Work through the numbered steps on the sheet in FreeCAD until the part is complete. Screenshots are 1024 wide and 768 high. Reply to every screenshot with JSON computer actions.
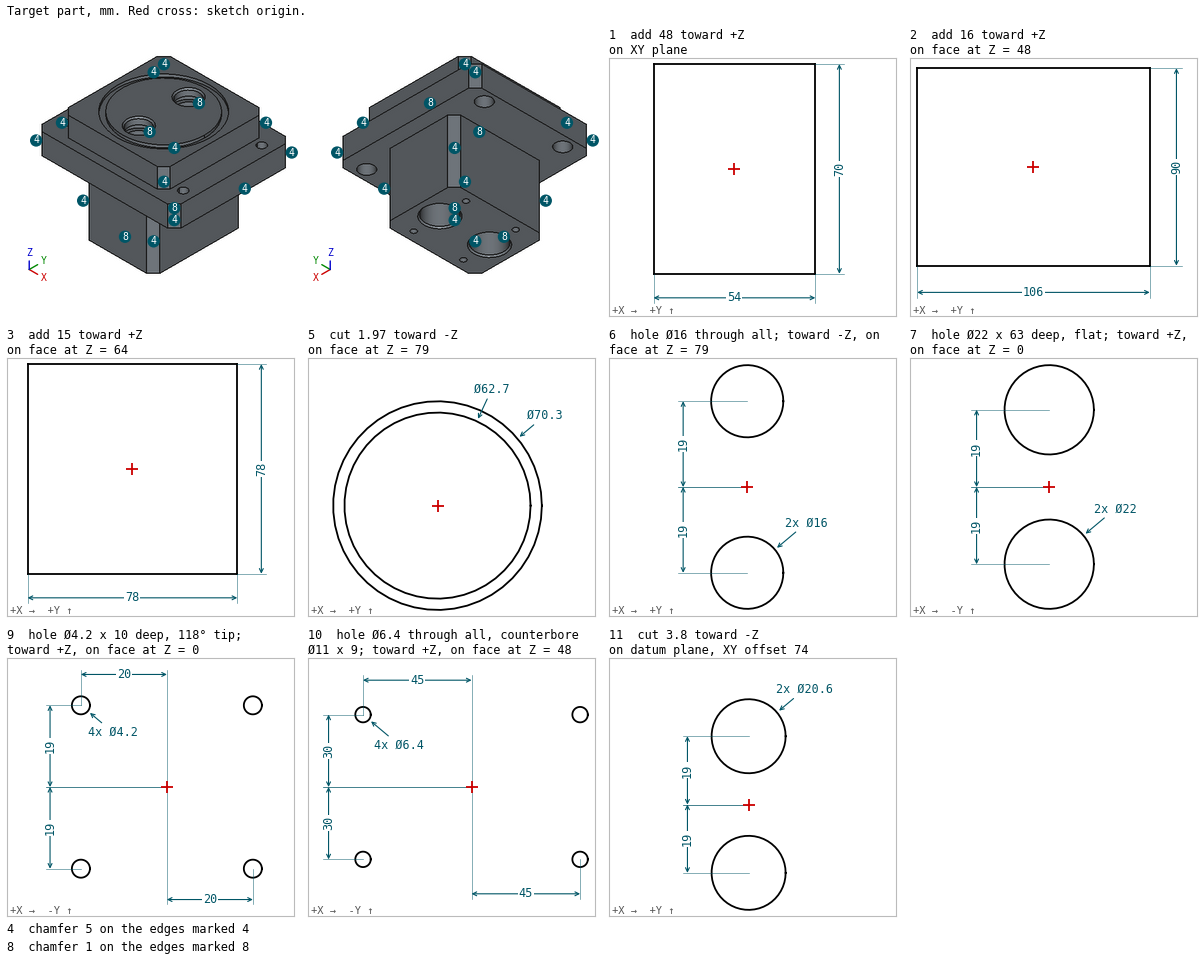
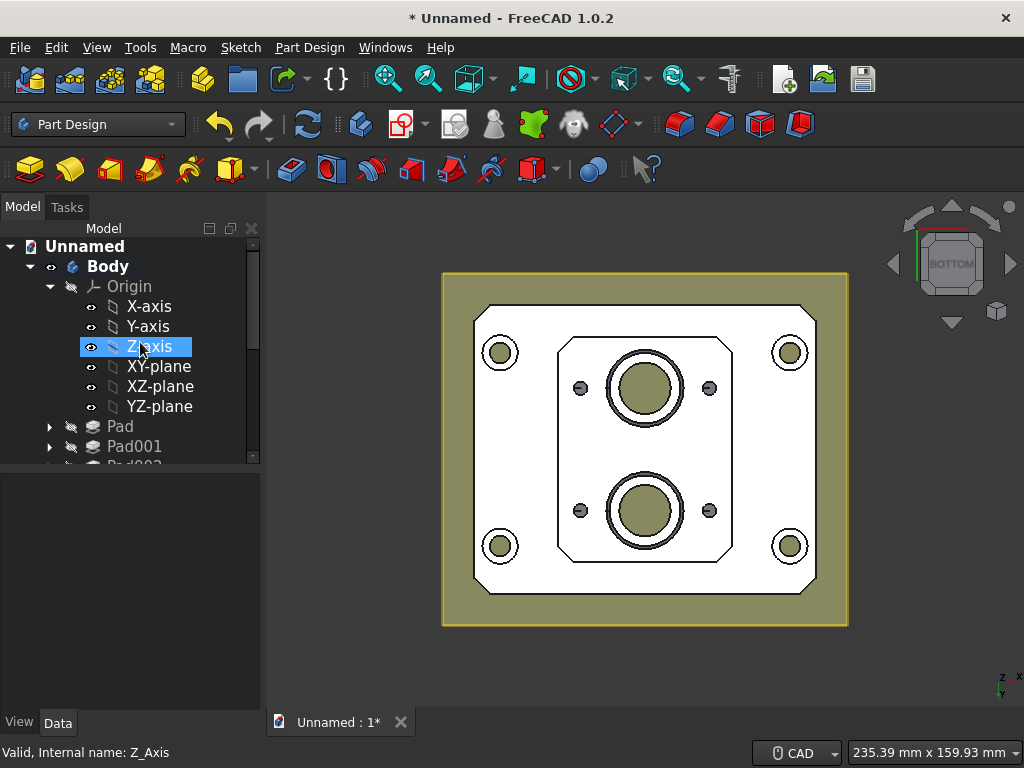
{"action": "scroll", "coordinate": [100, 342], "scroll_direction": "down", "scroll_amount": 6}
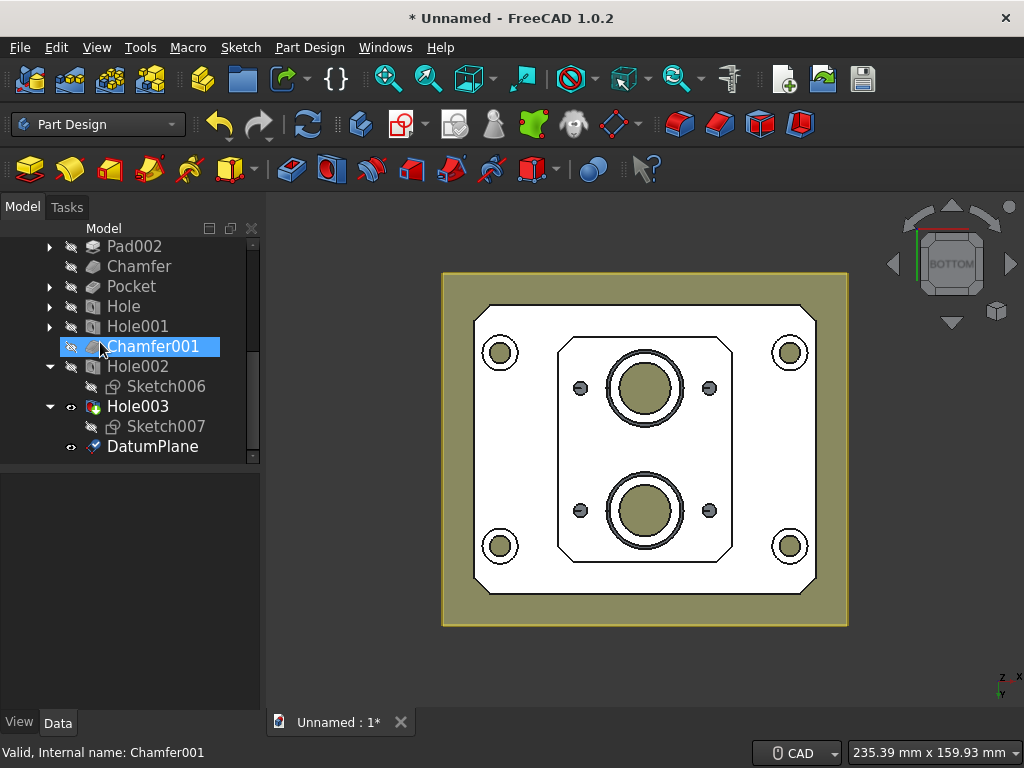
{"action": "left_click", "coordinate": [116, 447]}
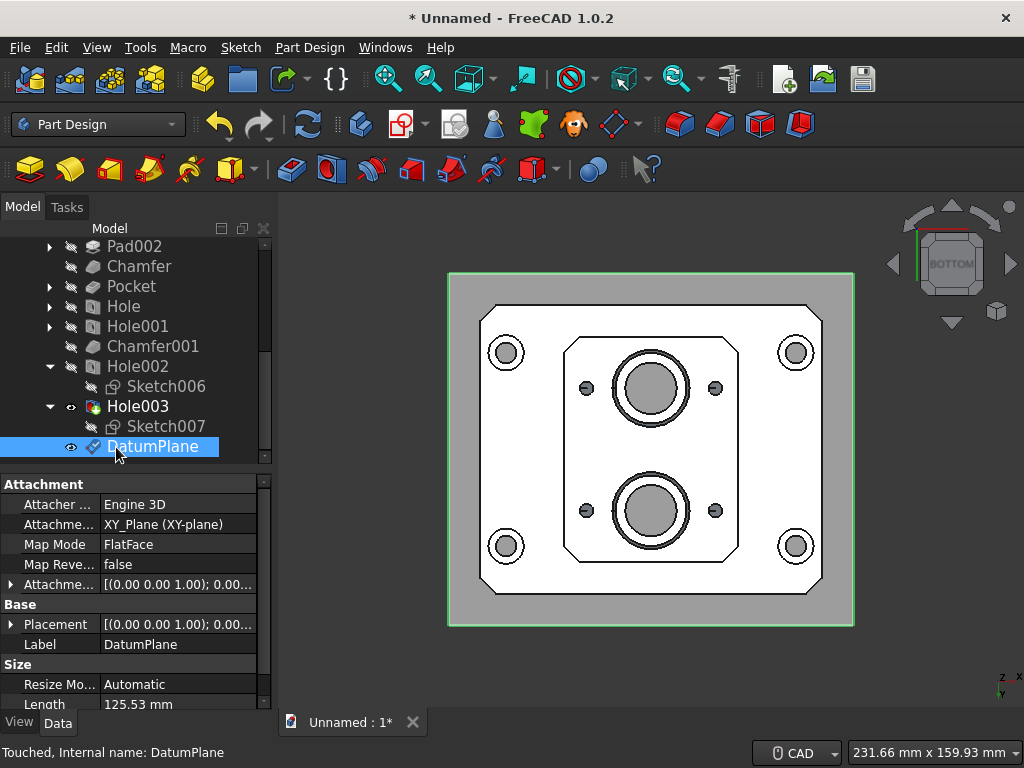
{"action": "left_click", "coordinate": [402, 124]}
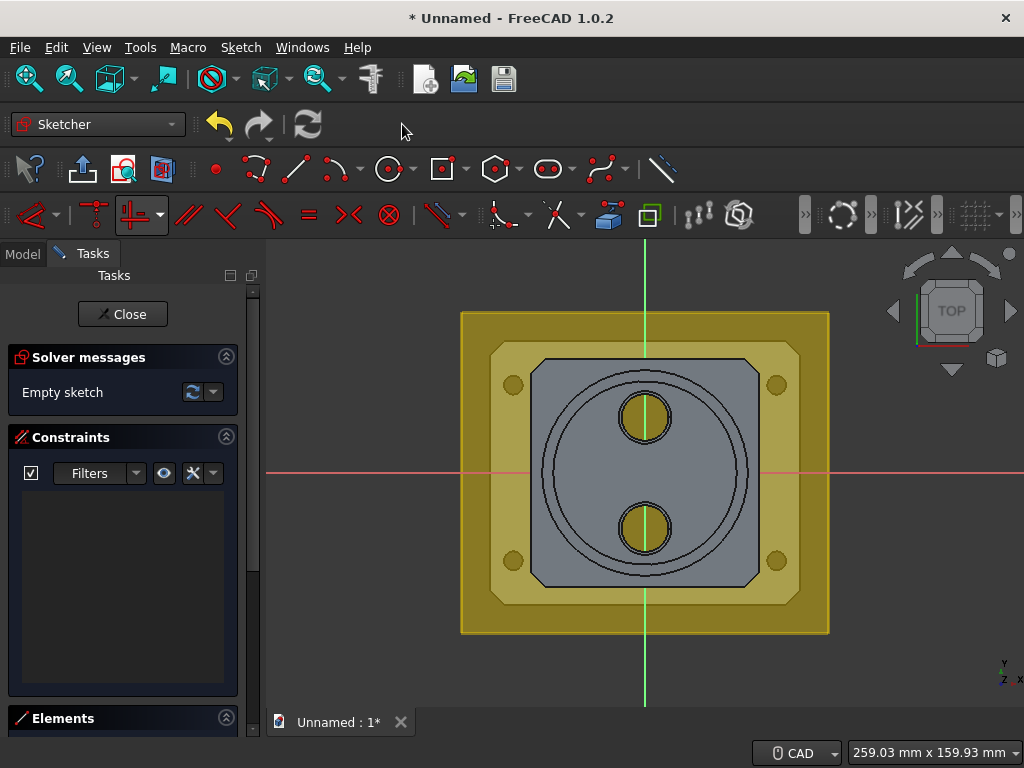
{"action": "left_click", "coordinate": [164, 170]}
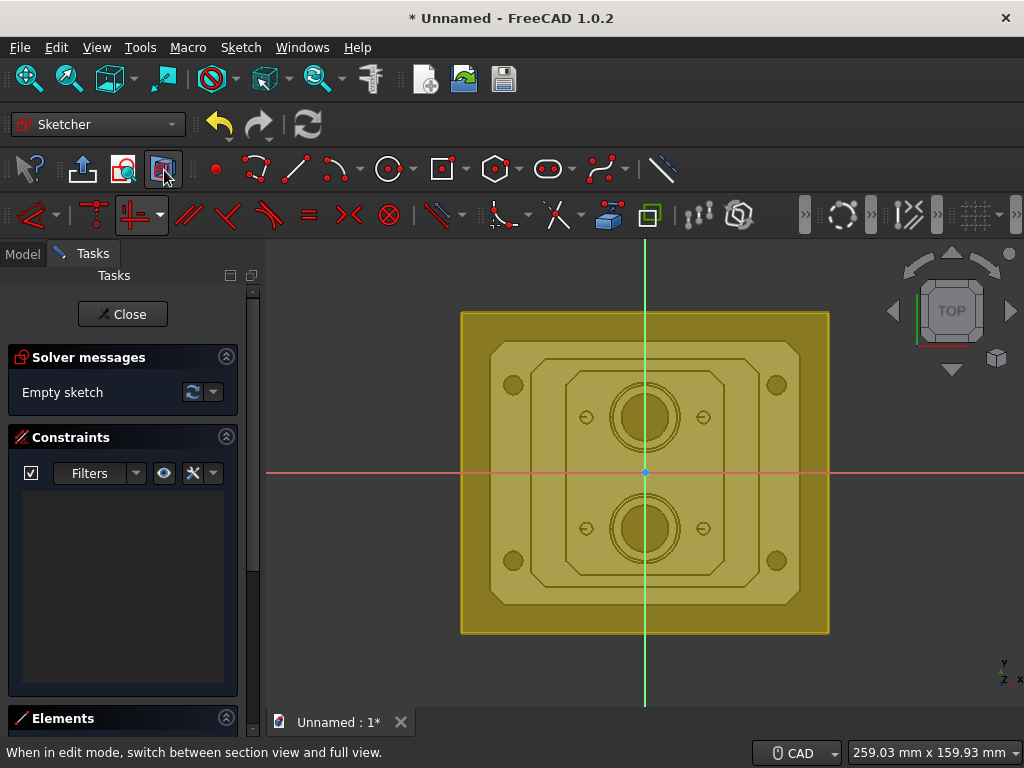
{"action": "scroll", "coordinate": [728, 473], "scroll_direction": "up", "scroll_amount": 3}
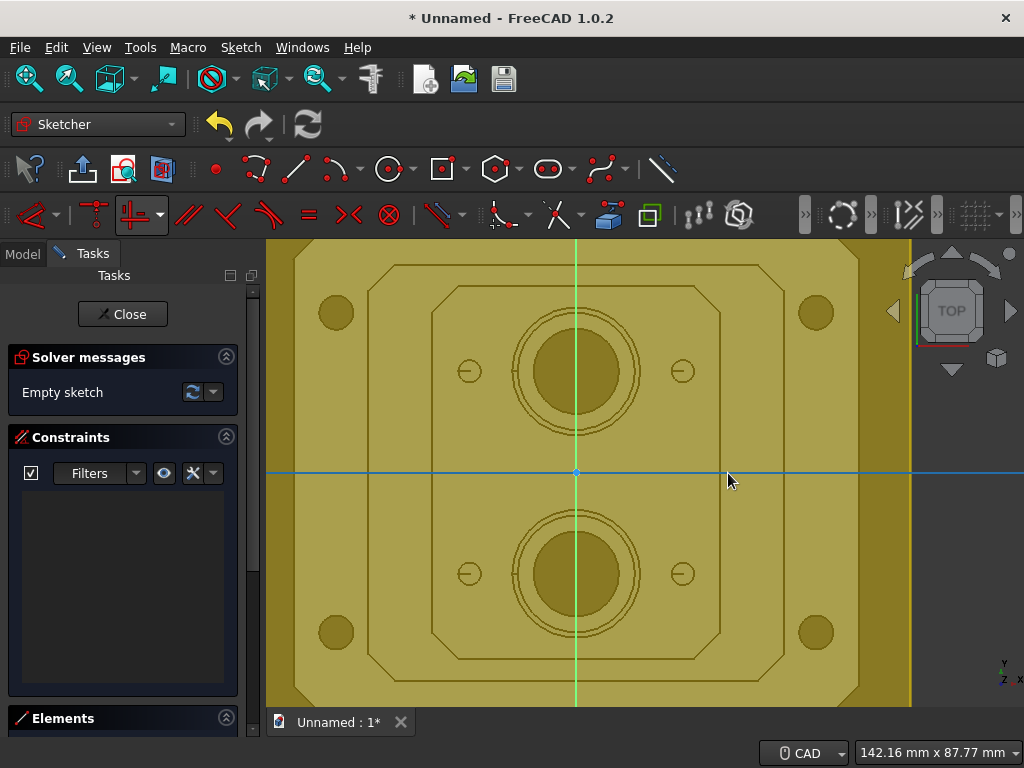
{"action": "left_click", "coordinate": [390, 170]}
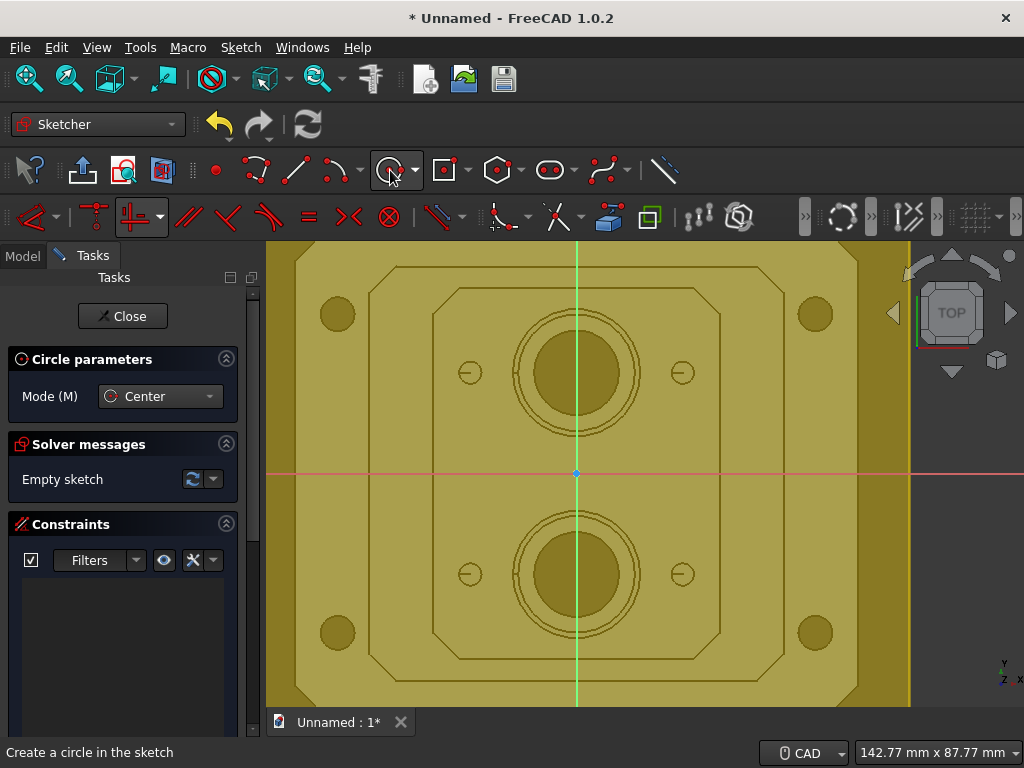
{"action": "left_click", "coordinate": [577, 373]}
{"action": "mouse_move", "coordinate": [615, 334]}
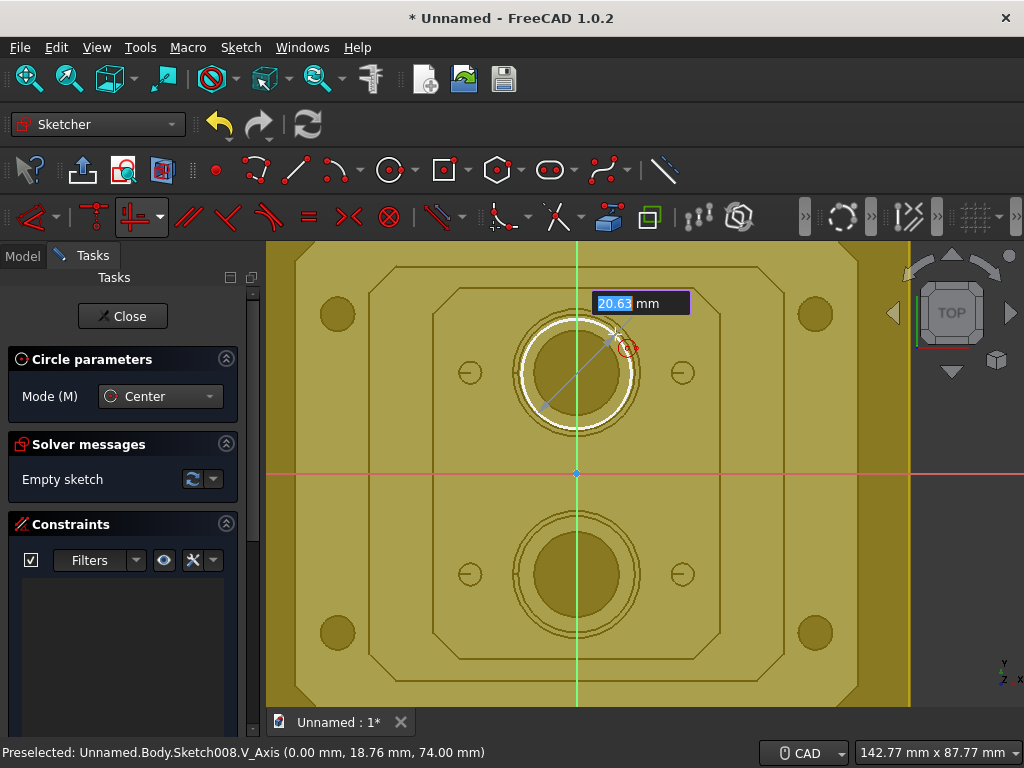
{"action": "type", "text": "20.6"}
{"action": "key", "text": "Return"}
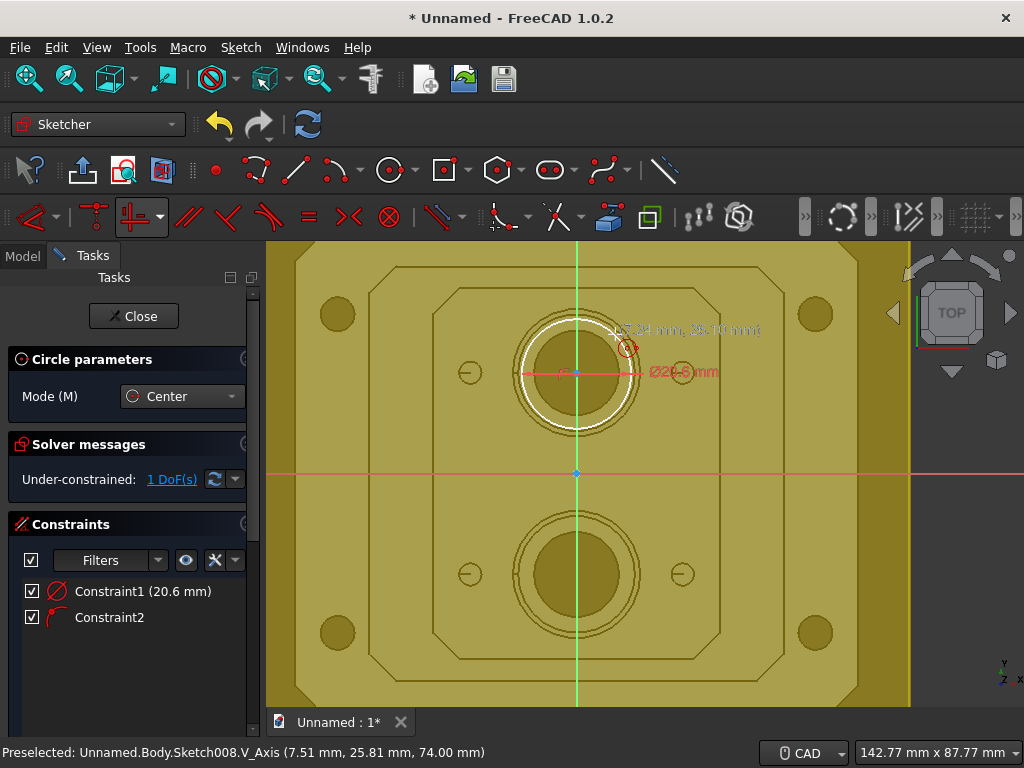
{"action": "left_click", "coordinate": [577, 574]}
{"action": "mouse_move", "coordinate": [615, 536]}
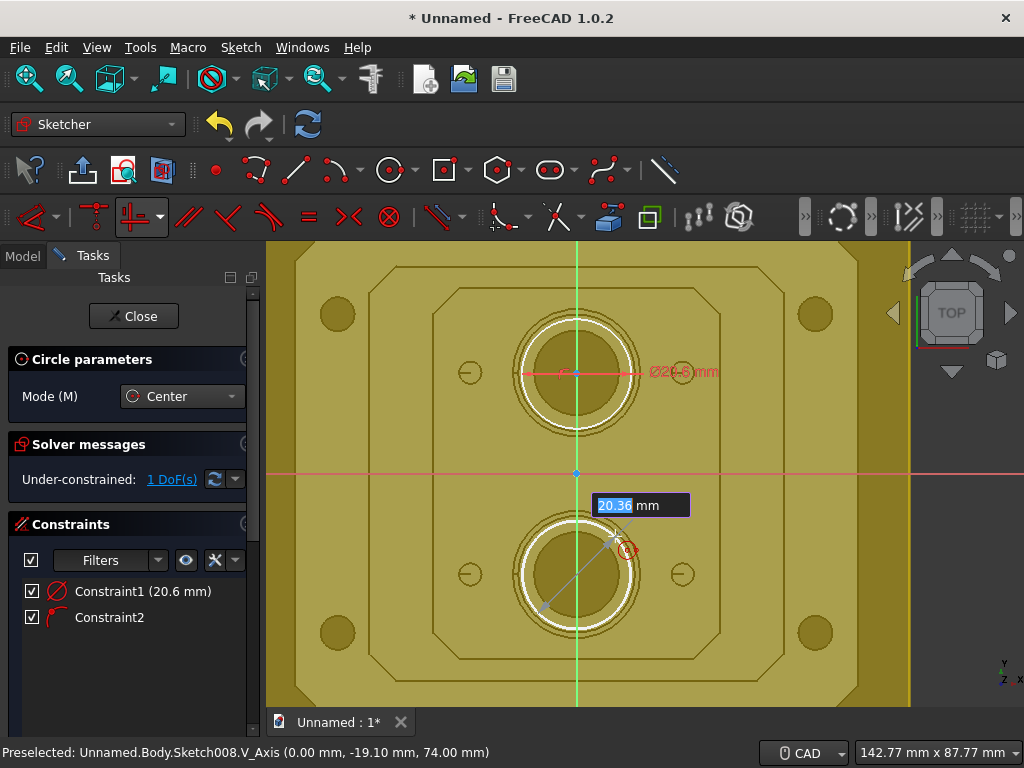
{"action": "type", "text": "20.6"}
{"action": "key", "text": "Return"}
{"action": "key", "text": "Escape"}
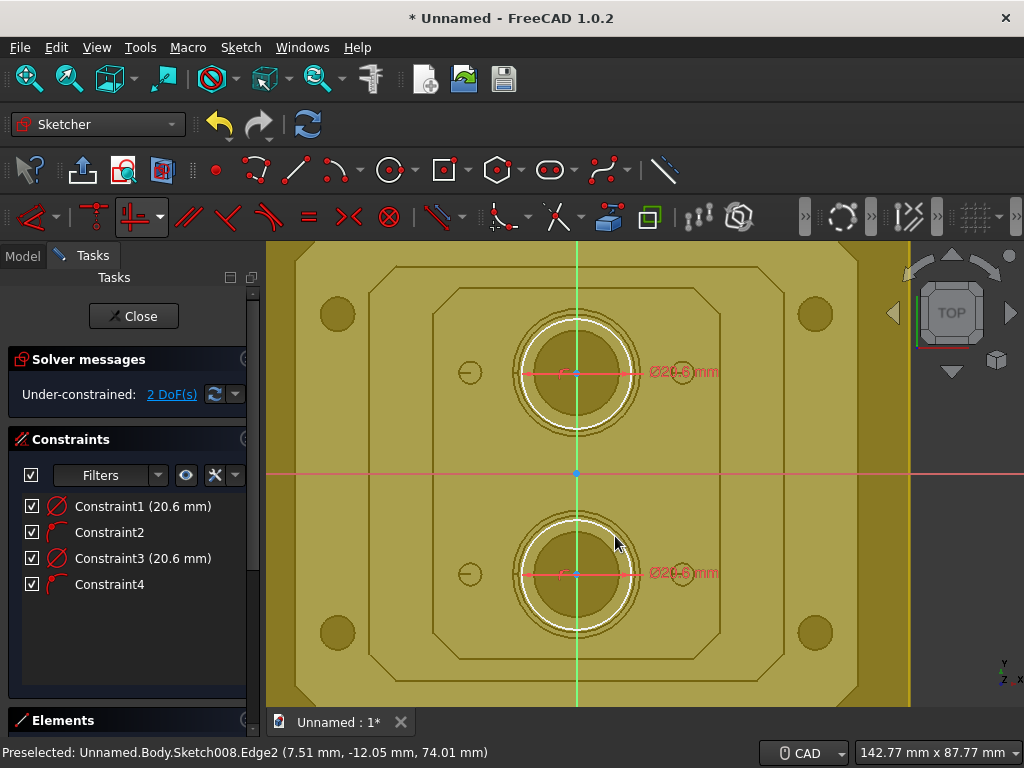
{"action": "left_click", "coordinate": [32, 218]}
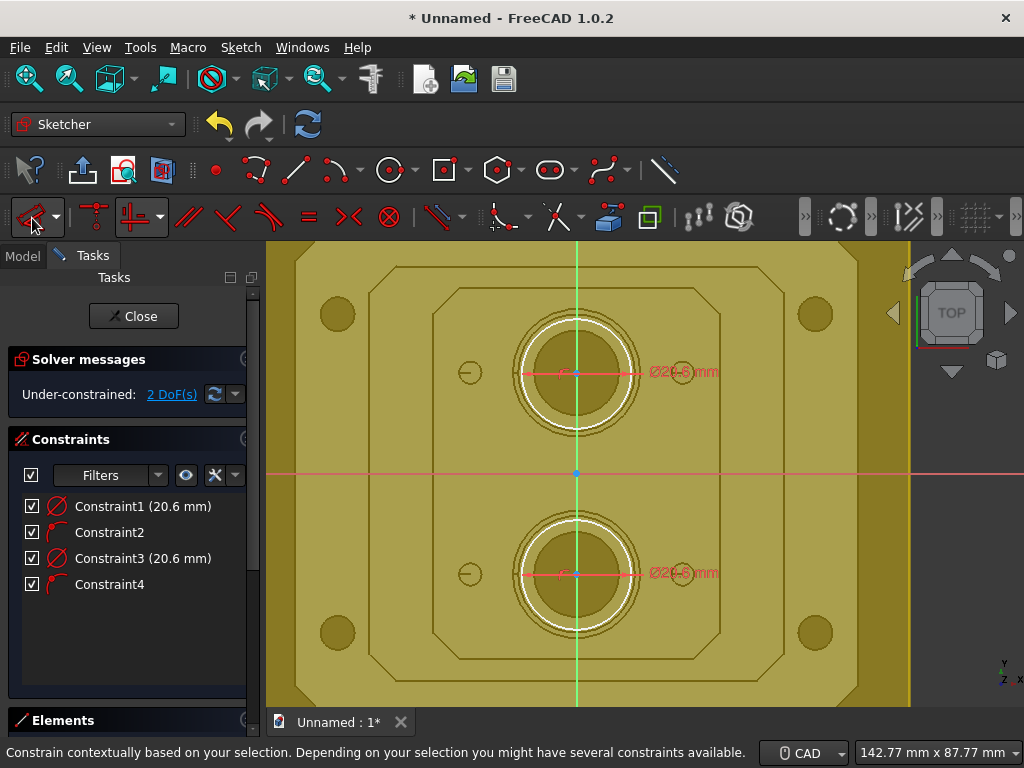
{"action": "left_click", "coordinate": [577, 374]}
{"action": "left_click", "coordinate": [611, 447]}